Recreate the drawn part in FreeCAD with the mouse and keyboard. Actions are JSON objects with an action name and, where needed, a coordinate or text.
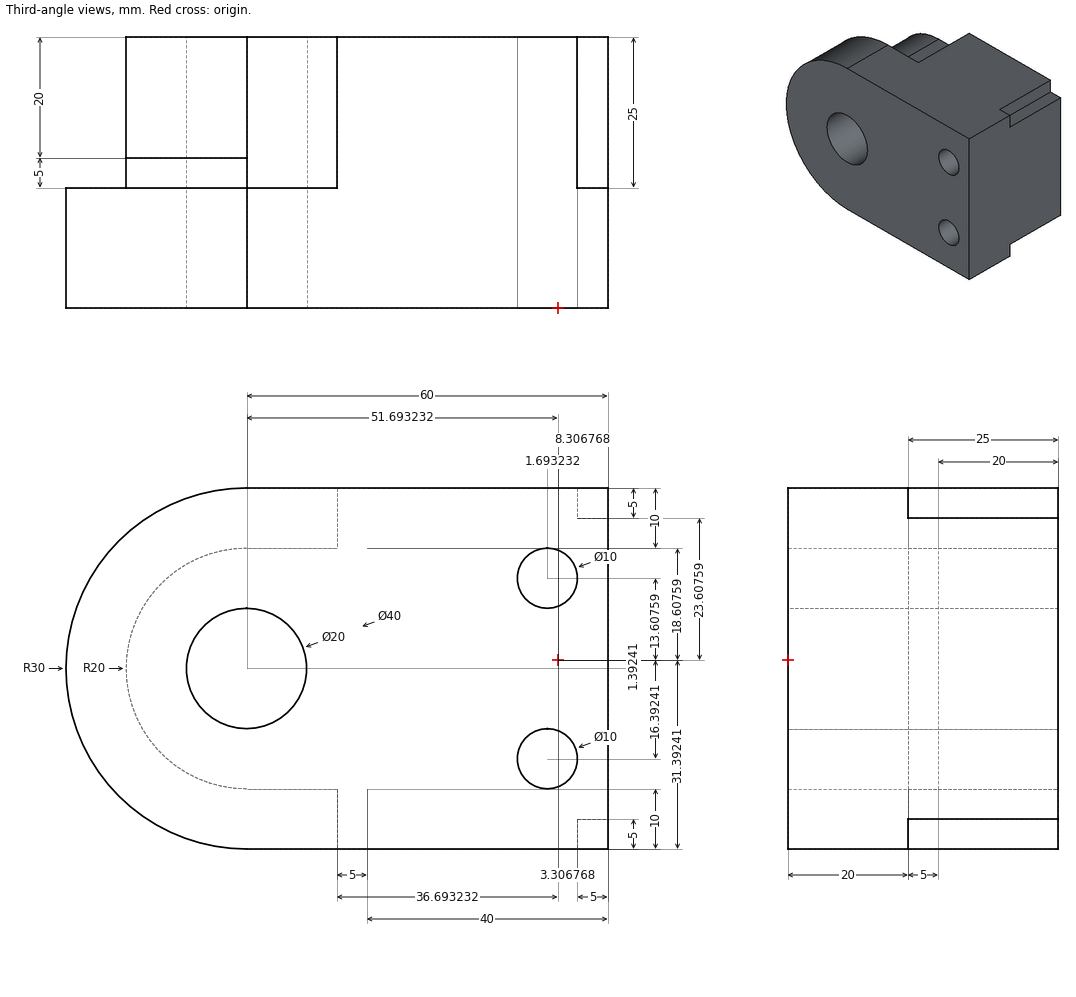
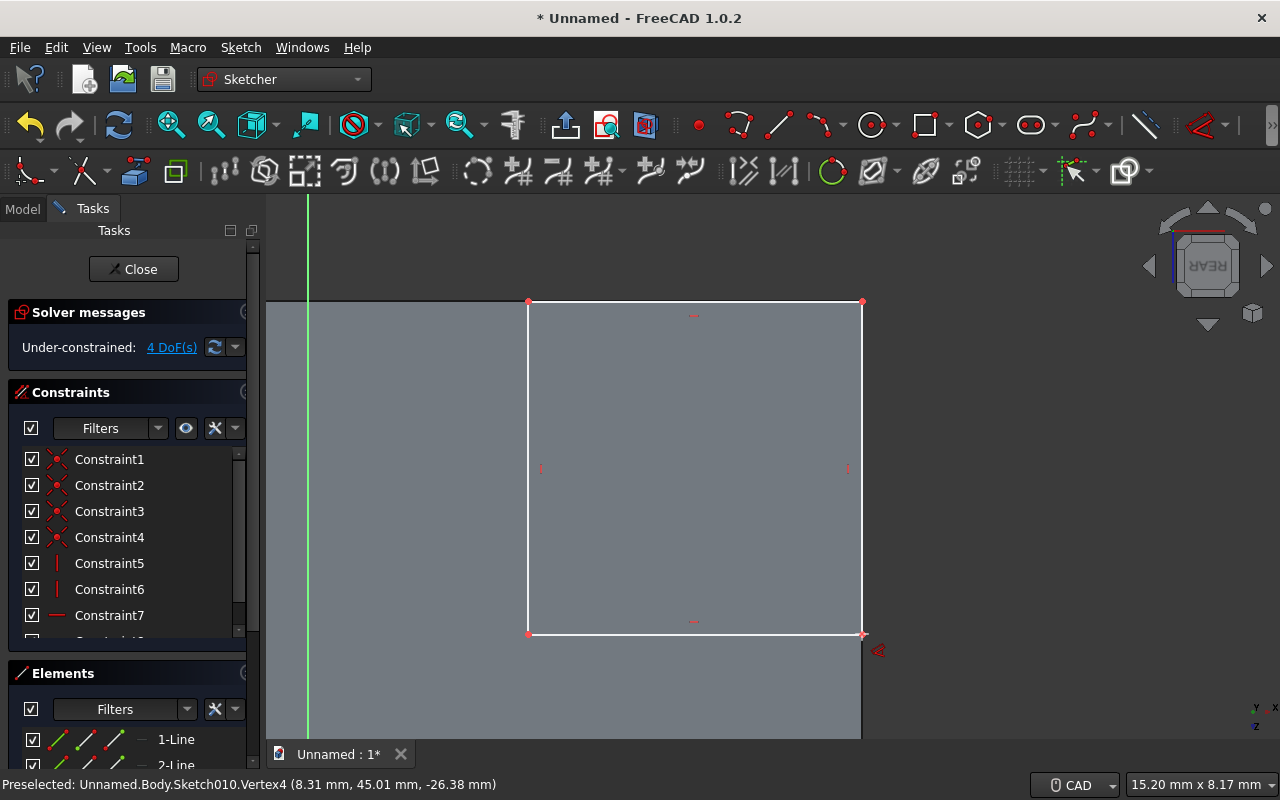
{"action": "left_click", "coordinate": [528, 402]}
{"action": "left_click", "coordinate": [494, 468]}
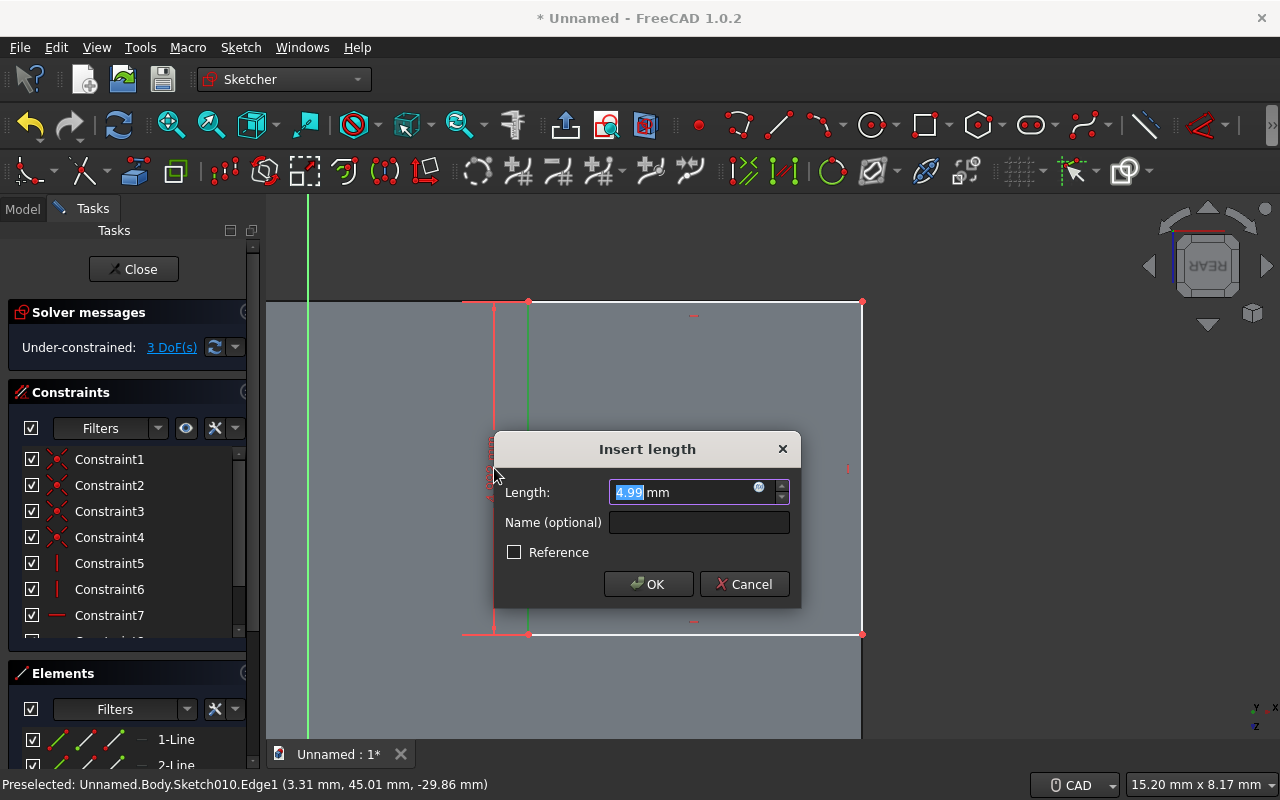
{"action": "type", "text": "5"}
{"action": "key", "text": "Return"}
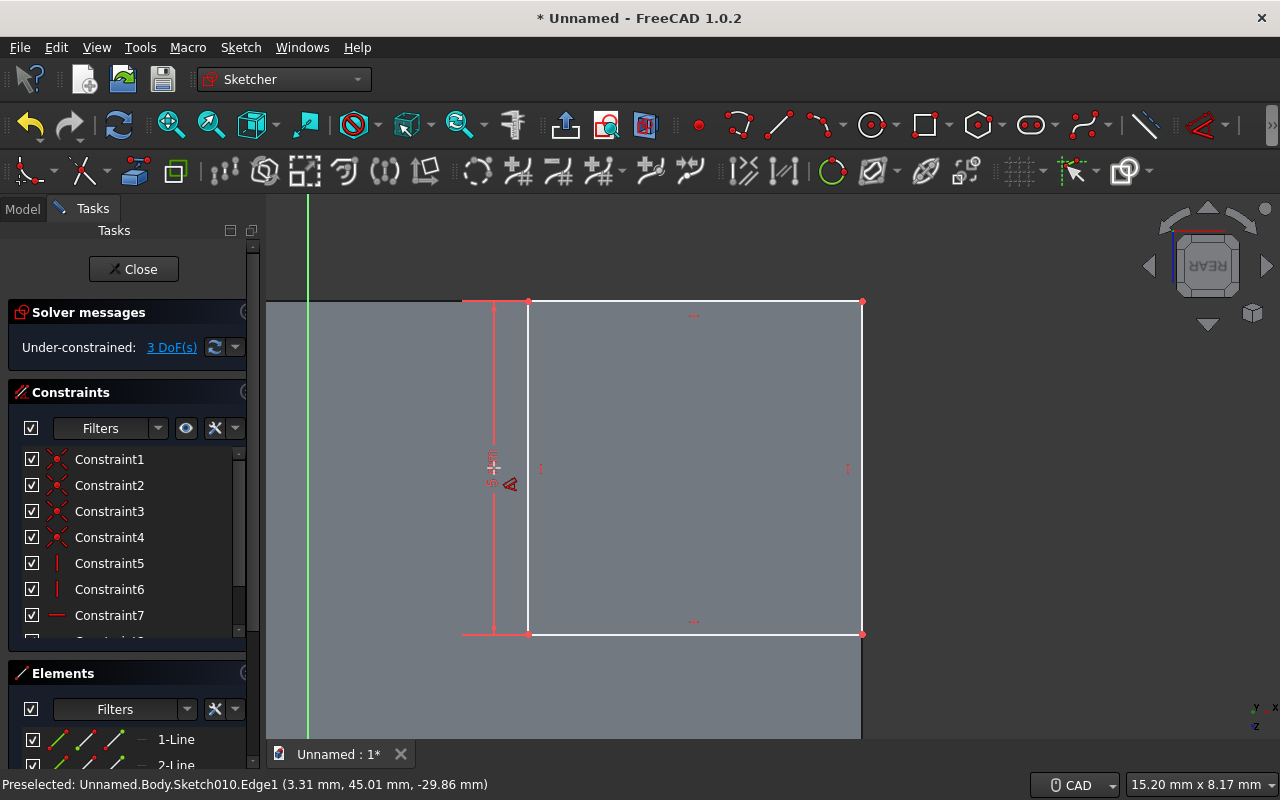
{"action": "left_click", "coordinate": [628, 635]}
{"action": "left_click", "coordinate": [695, 669]}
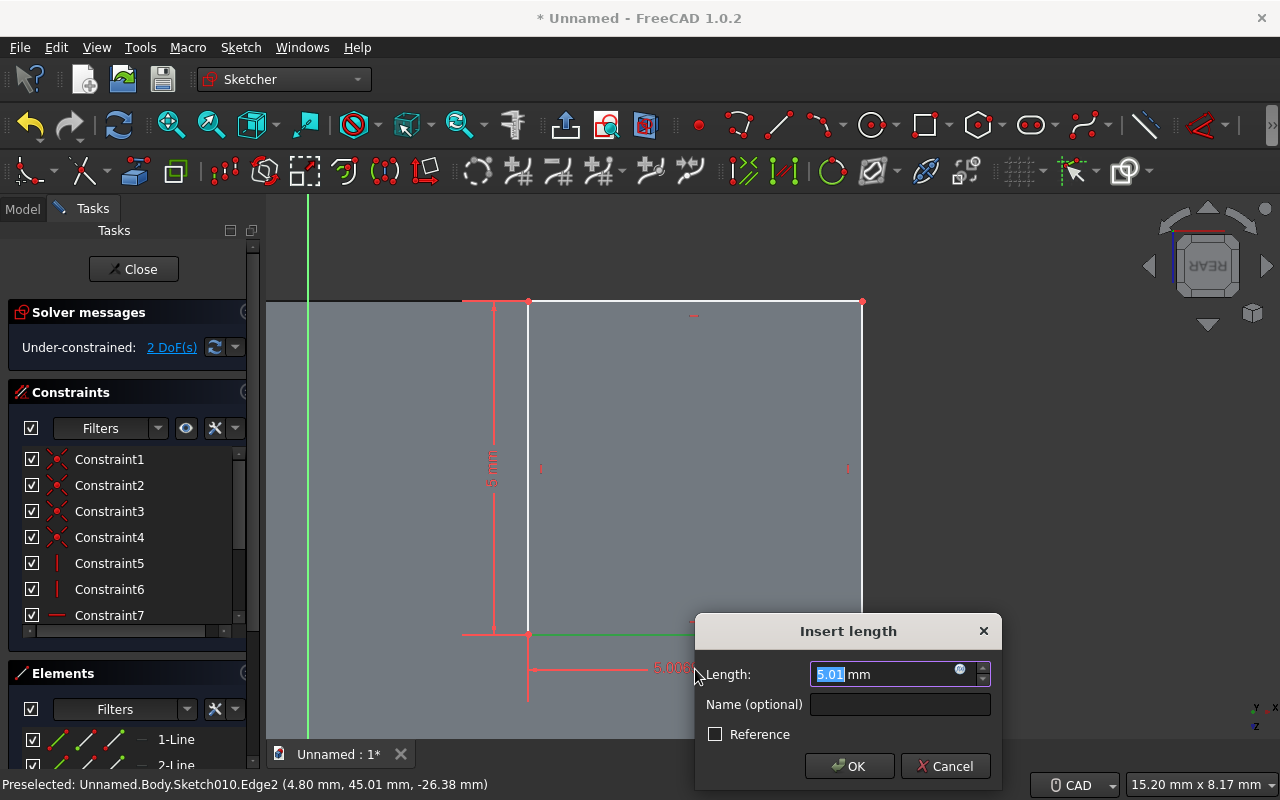
{"action": "type", "text": "5"}
{"action": "key", "text": "Return"}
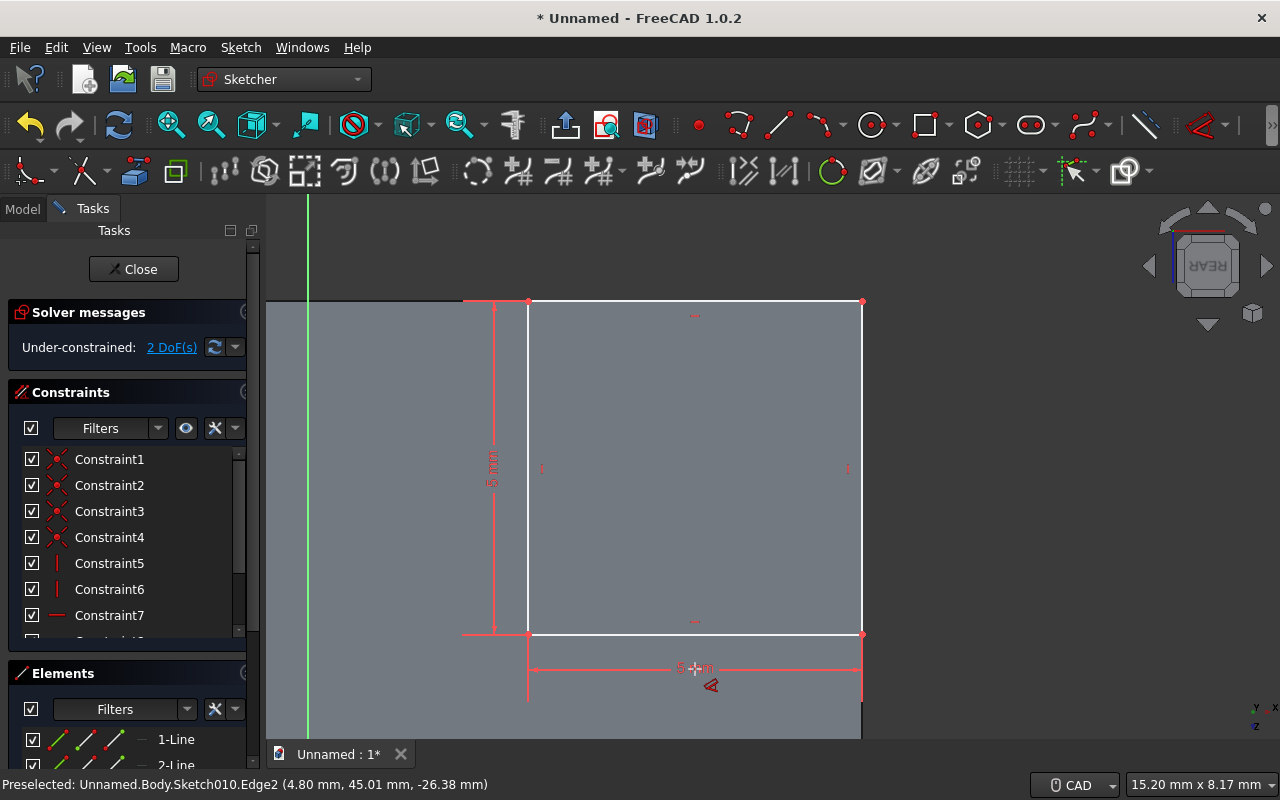
{"action": "left_click", "coordinate": [528, 301]}
{"action": "left_click", "coordinate": [418, 267]}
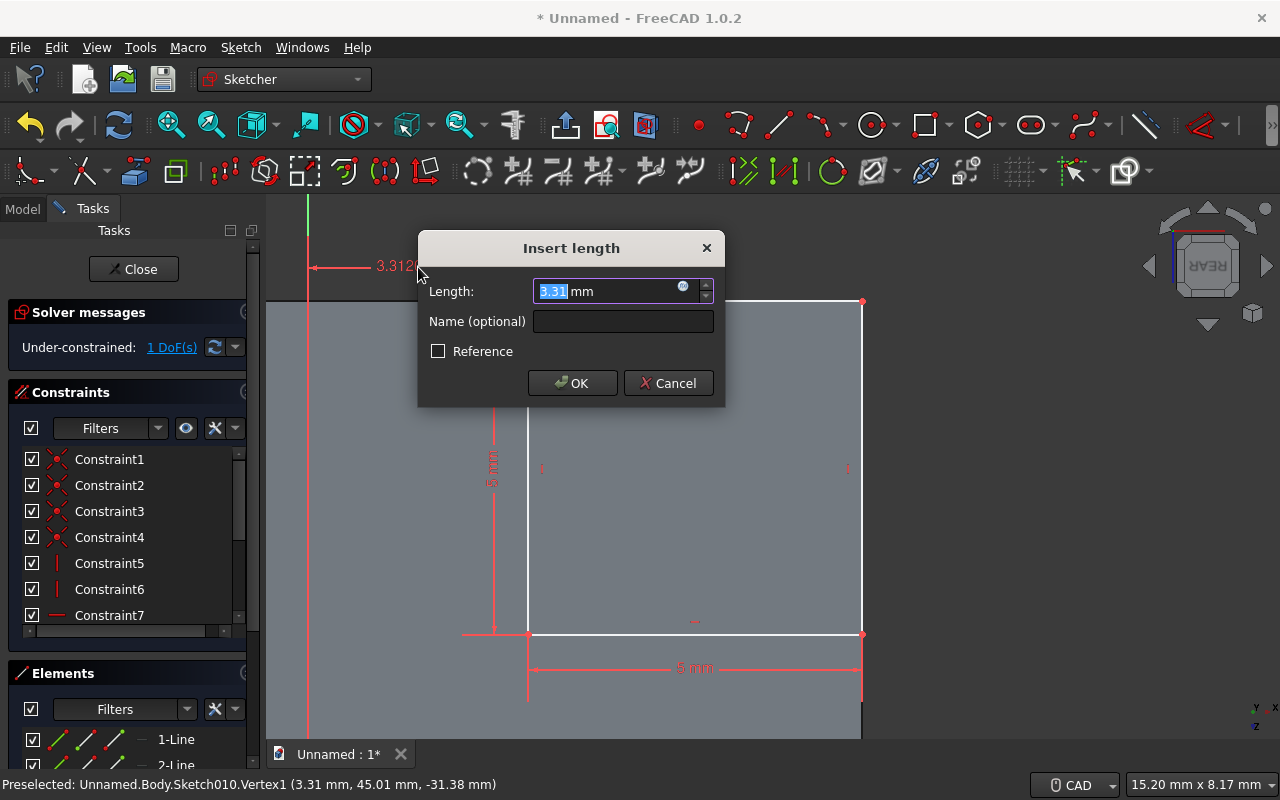
{"action": "type", "text": "3.306768"}
{"action": "key", "text": "Return"}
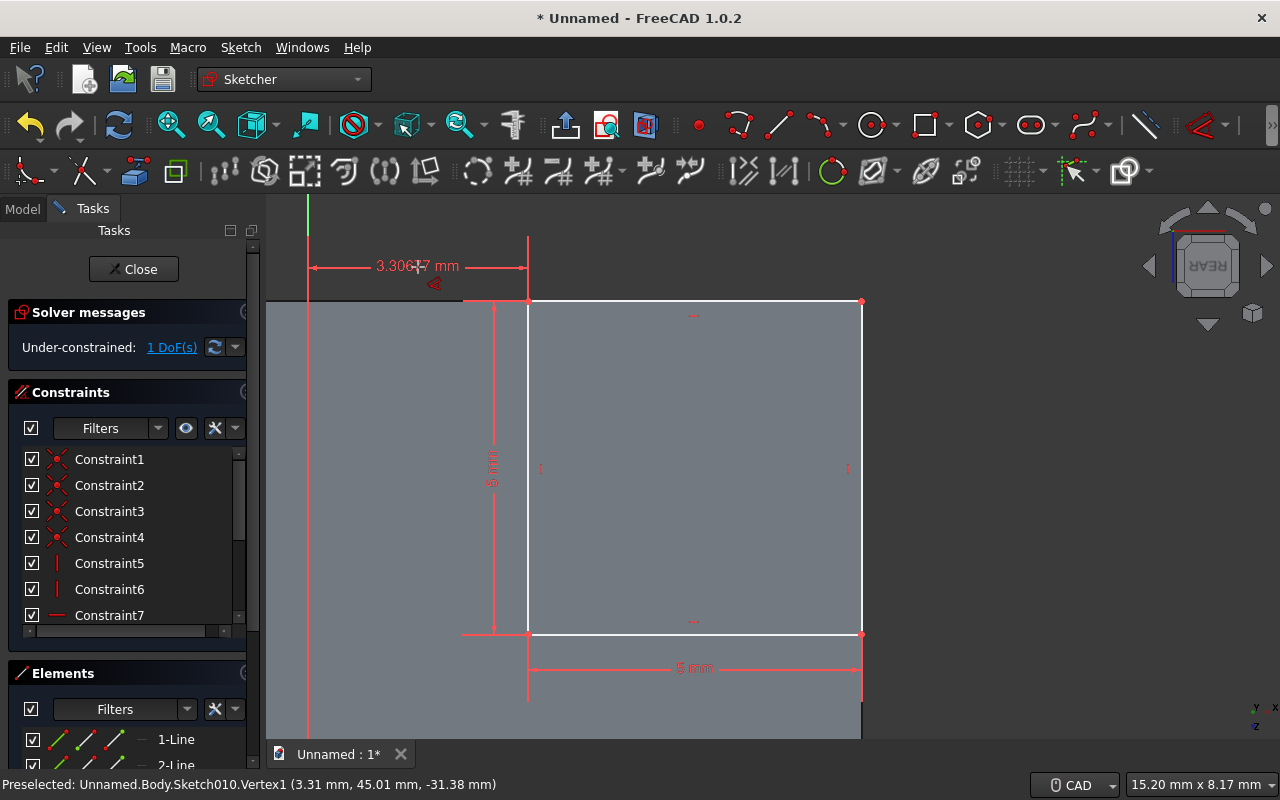
{"action": "left_click", "coordinate": [528, 301]}
{"action": "left_click", "coordinate": [562, 506]}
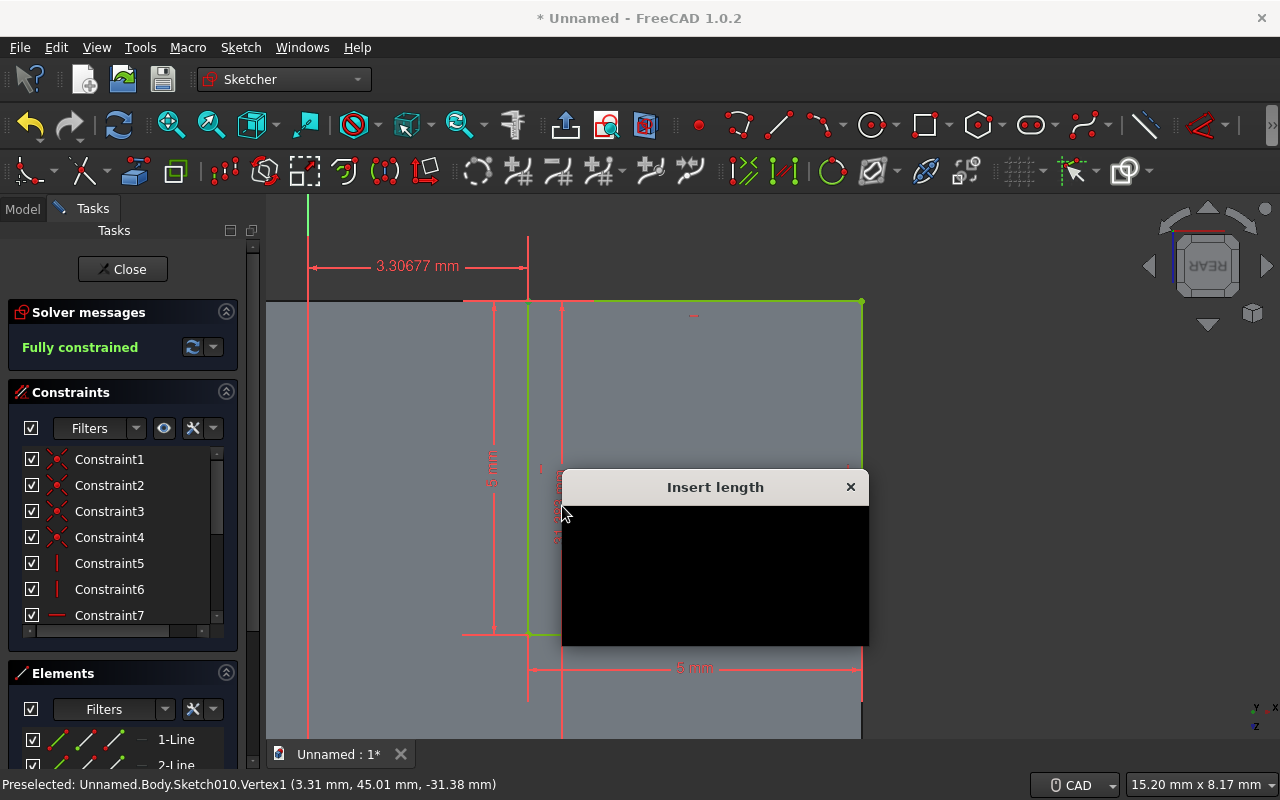
{"action": "type", "text": "31.39241"}
{"action": "key", "text": "Return"}
{"action": "key", "text": "Escape"}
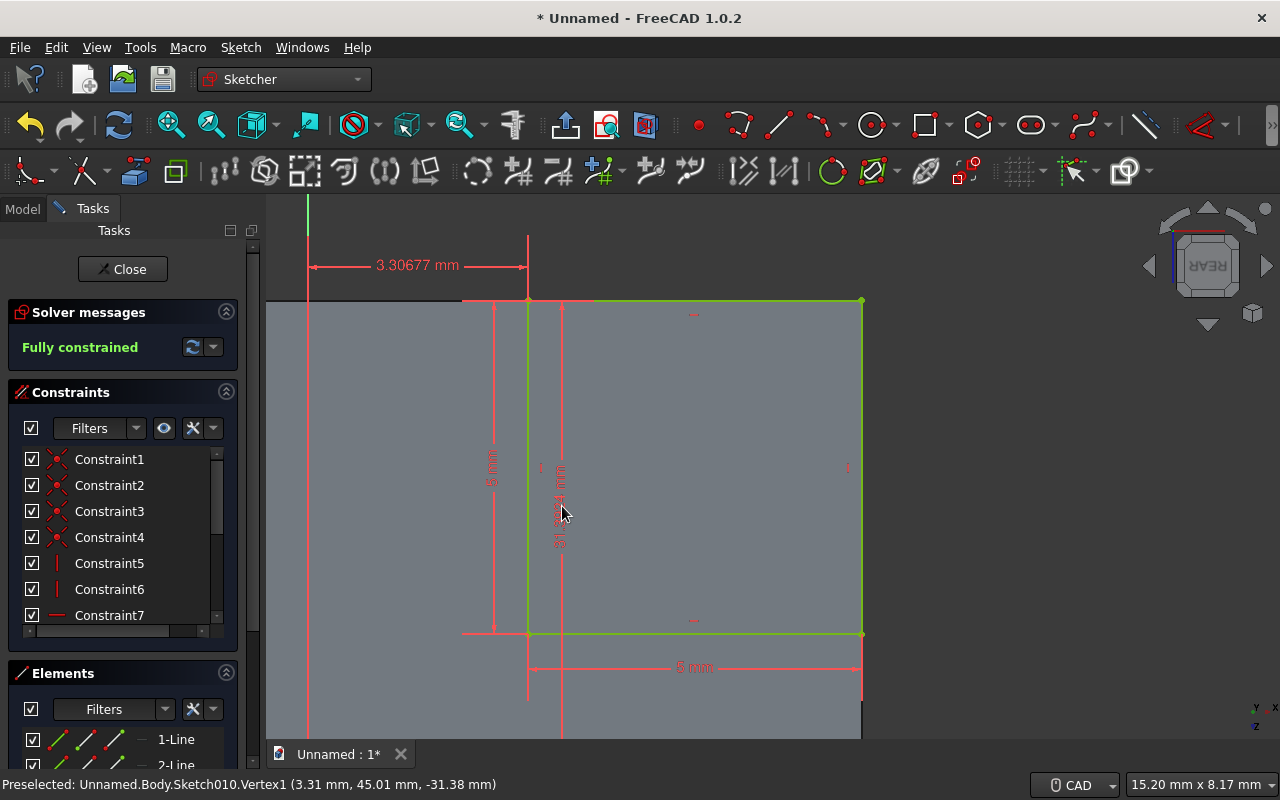
{"action": "left_click", "coordinate": [123, 269]}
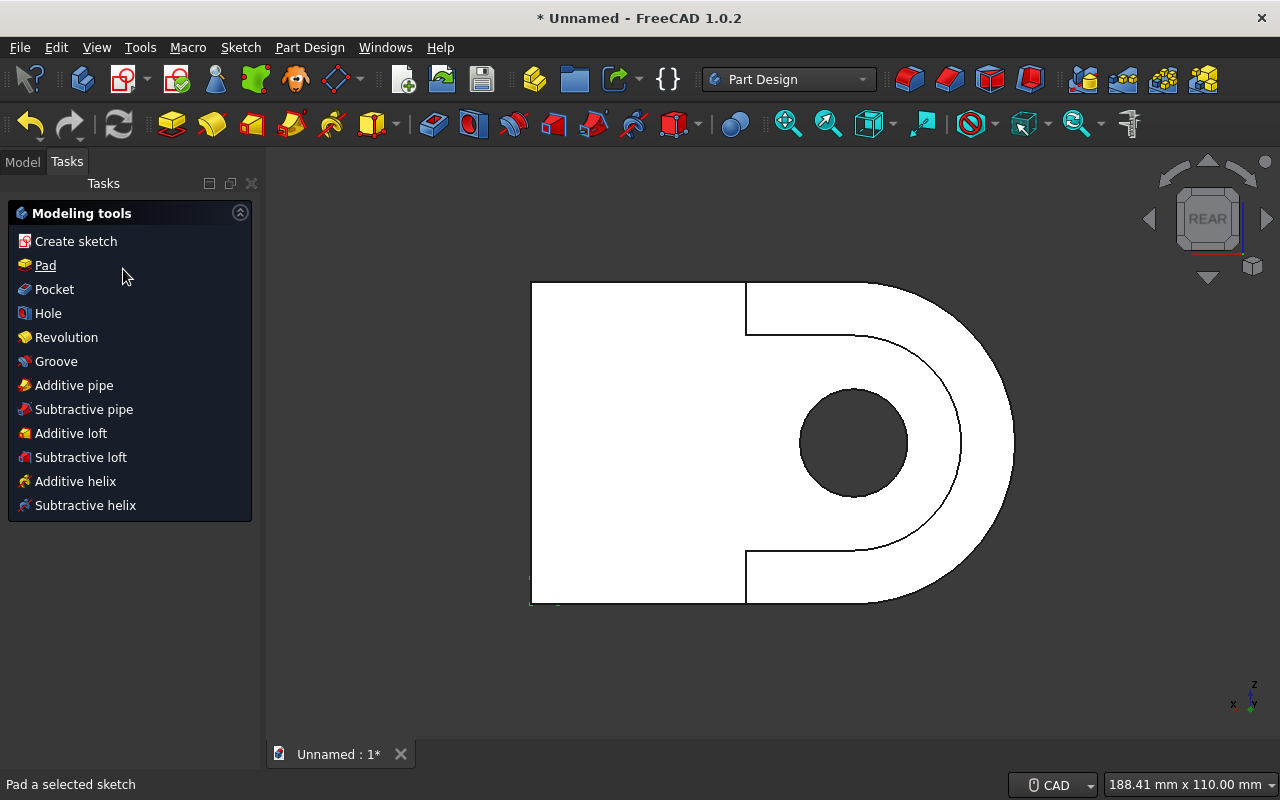
{"action": "left_click", "coordinate": [434, 124]}